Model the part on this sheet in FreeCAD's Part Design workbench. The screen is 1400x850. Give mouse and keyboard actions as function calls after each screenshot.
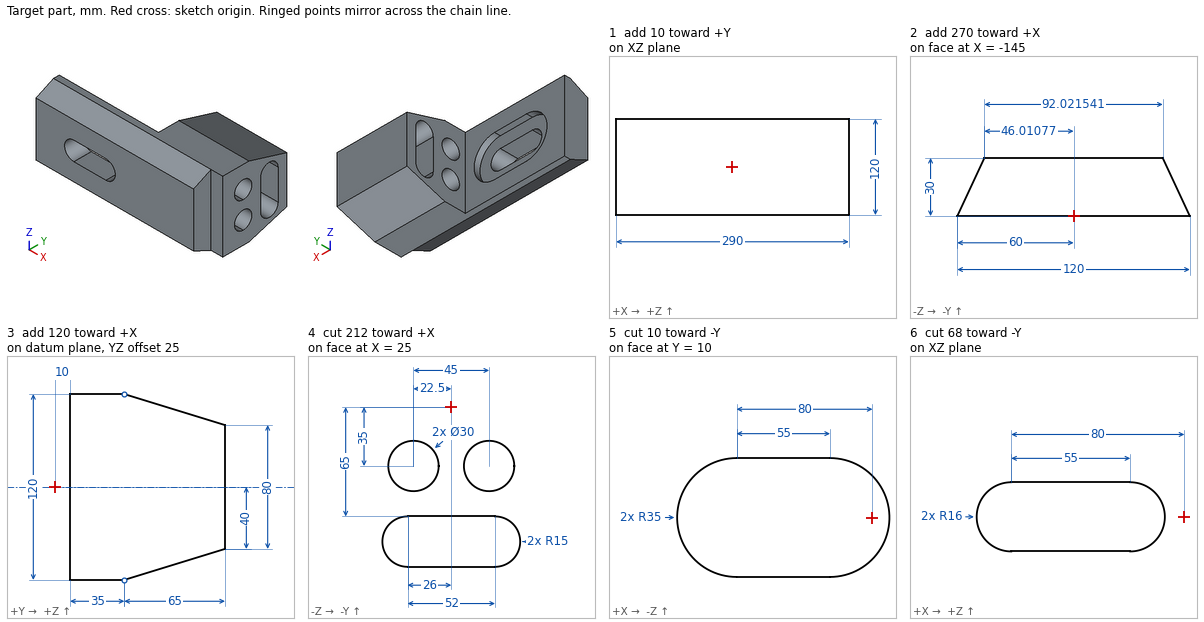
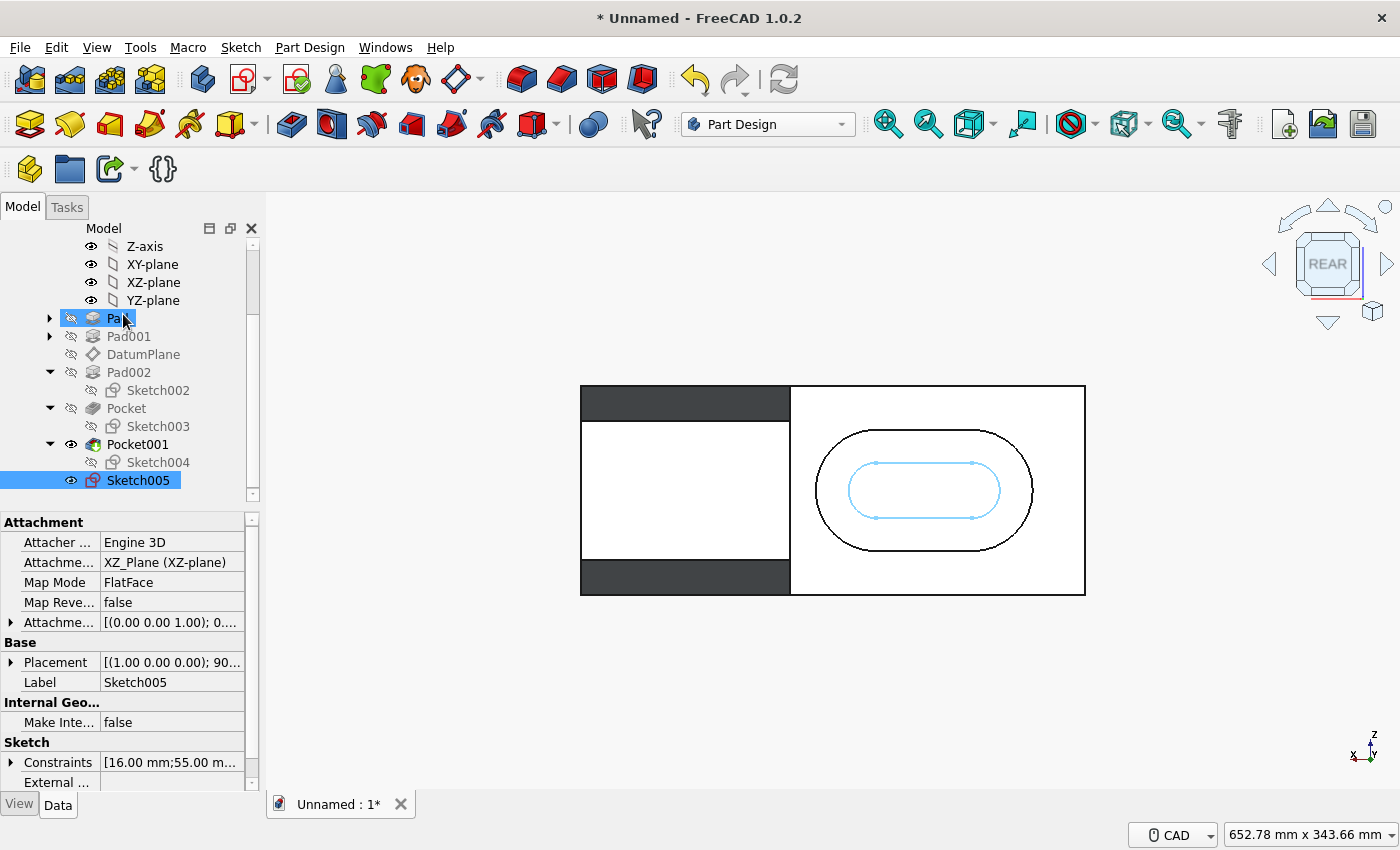
click(292, 124)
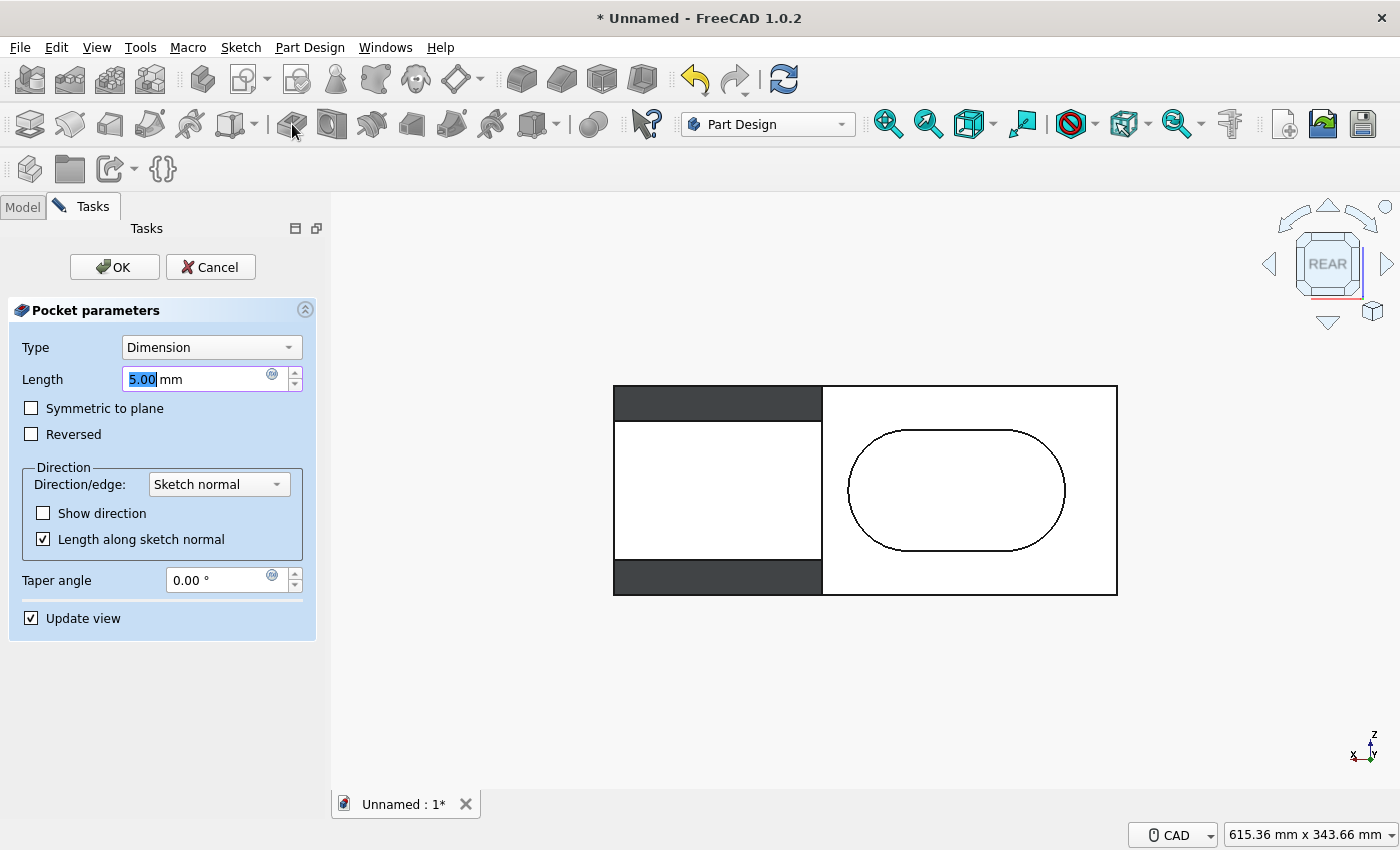
text(68)
key(Tab)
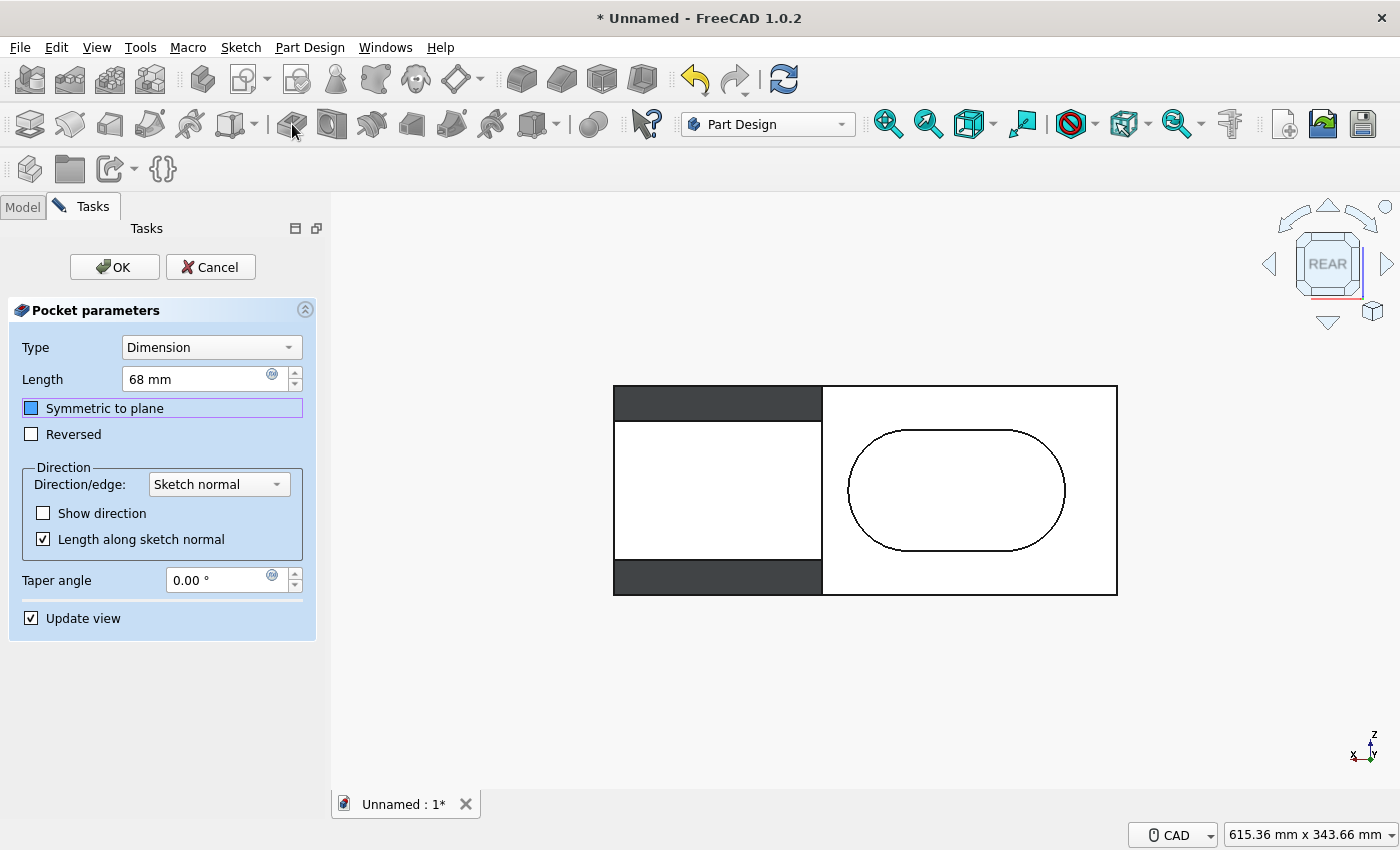
click(30, 434)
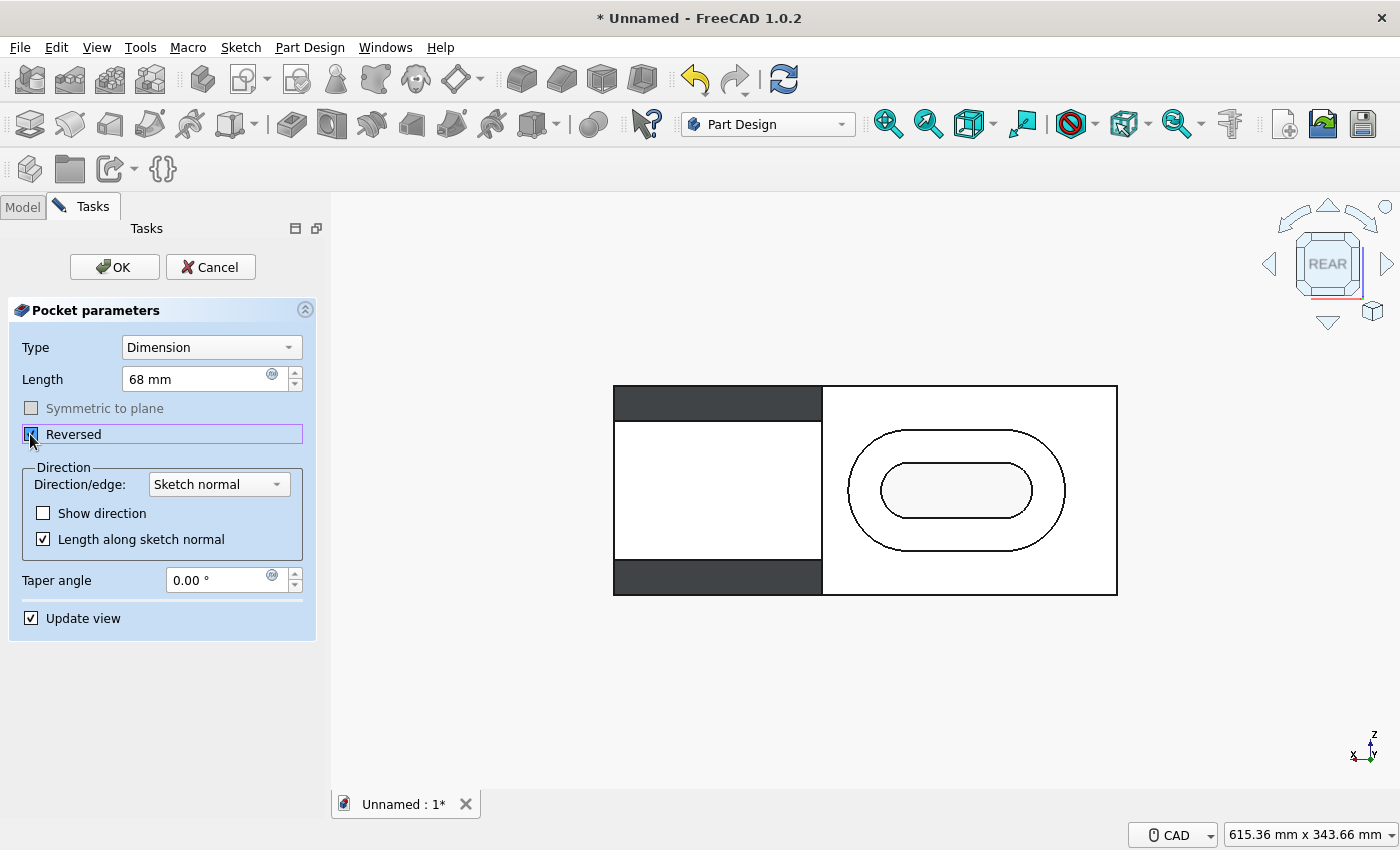
click(115, 267)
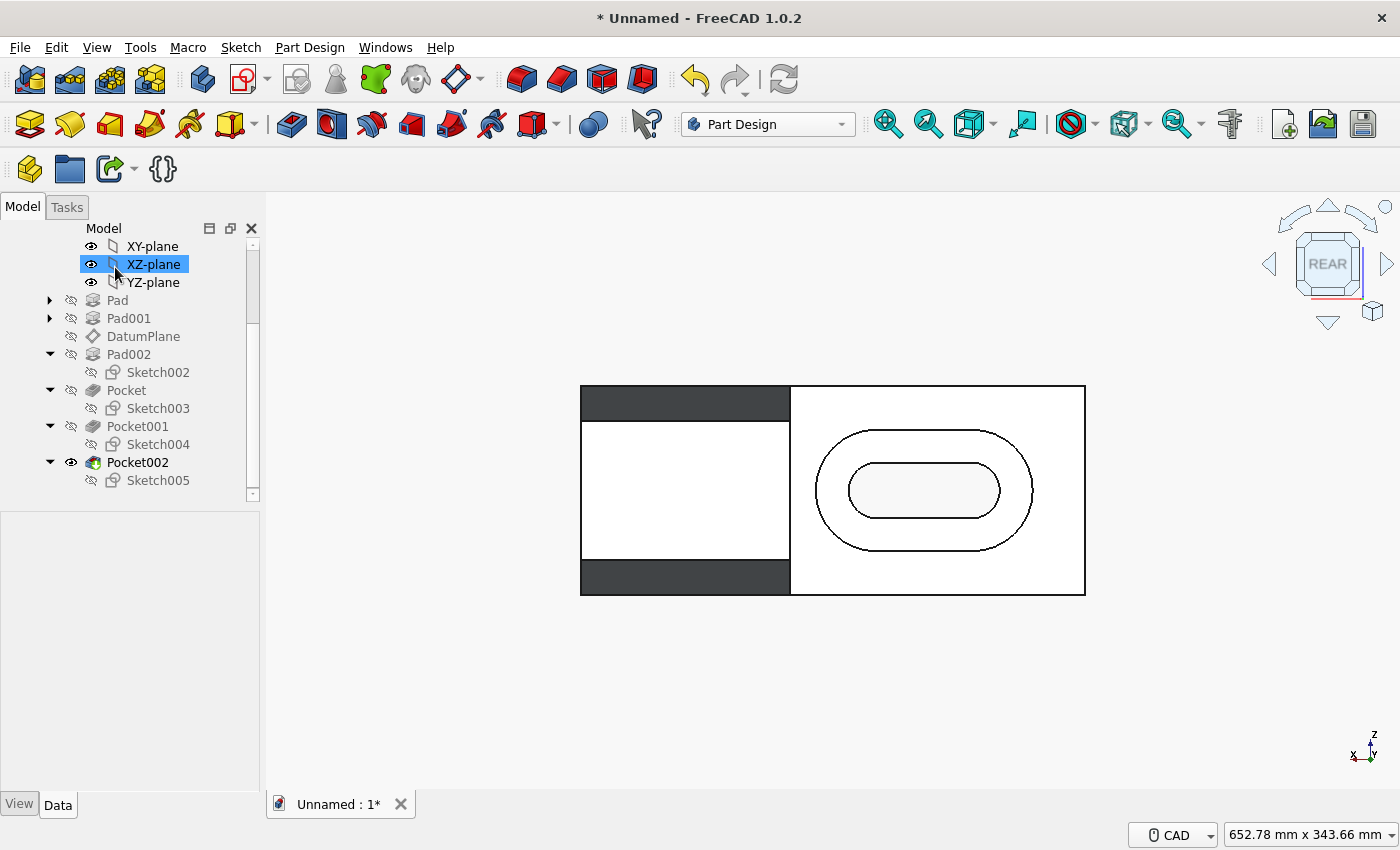
key(0)